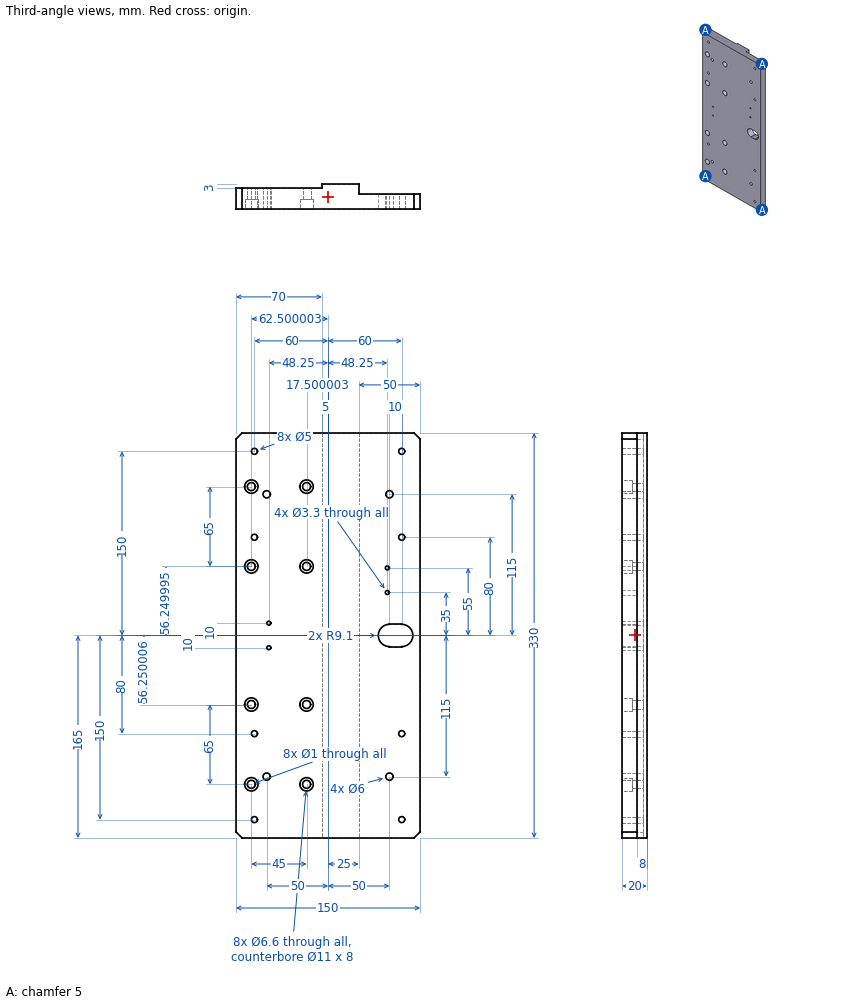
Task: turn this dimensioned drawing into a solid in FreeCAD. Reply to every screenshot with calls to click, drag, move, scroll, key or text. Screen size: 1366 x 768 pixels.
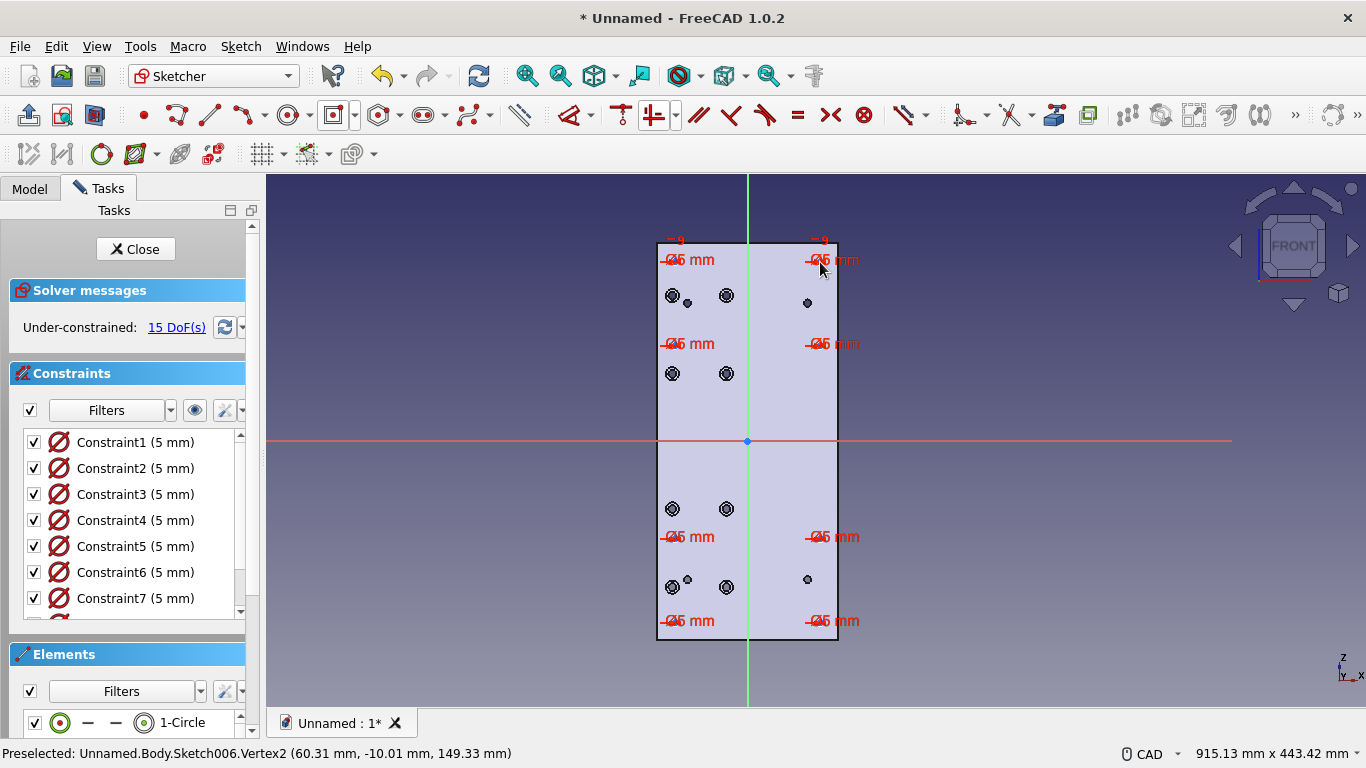
click(820, 262)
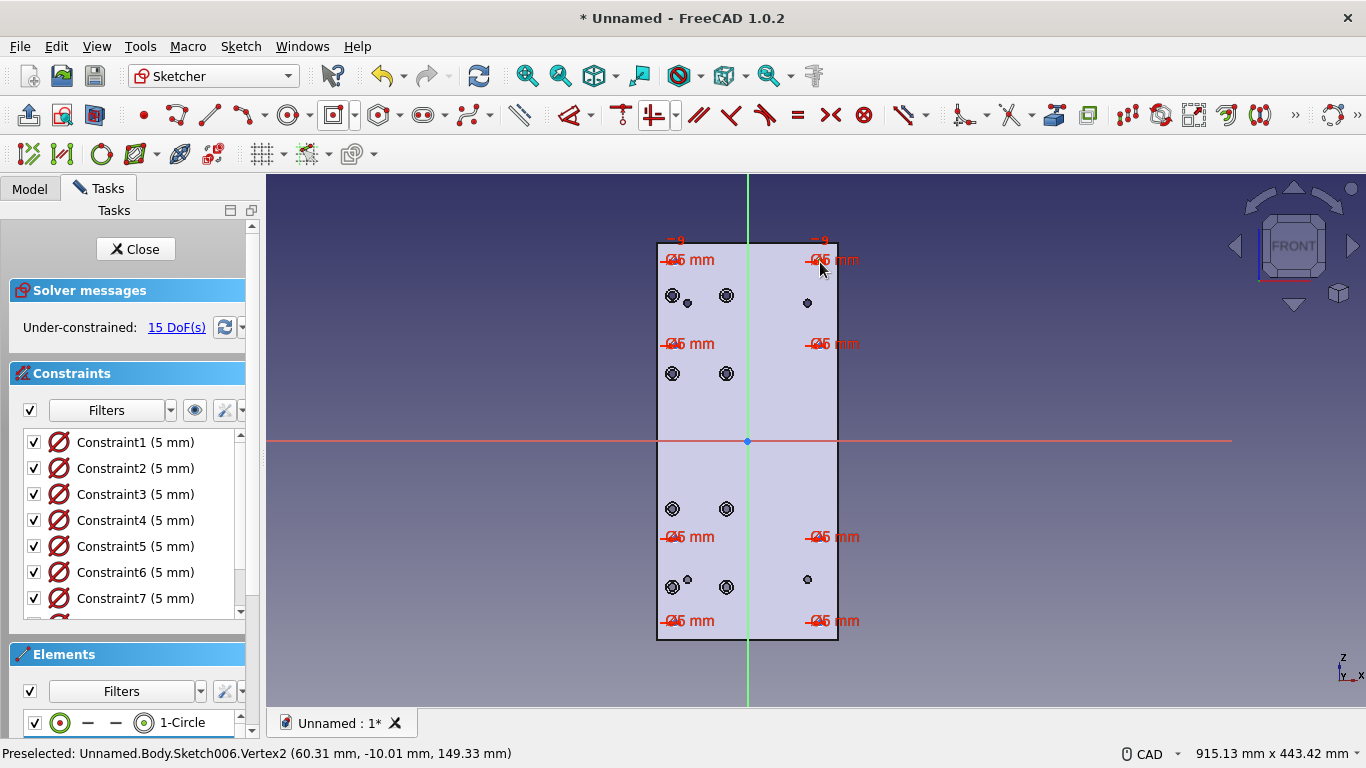
click(820, 346)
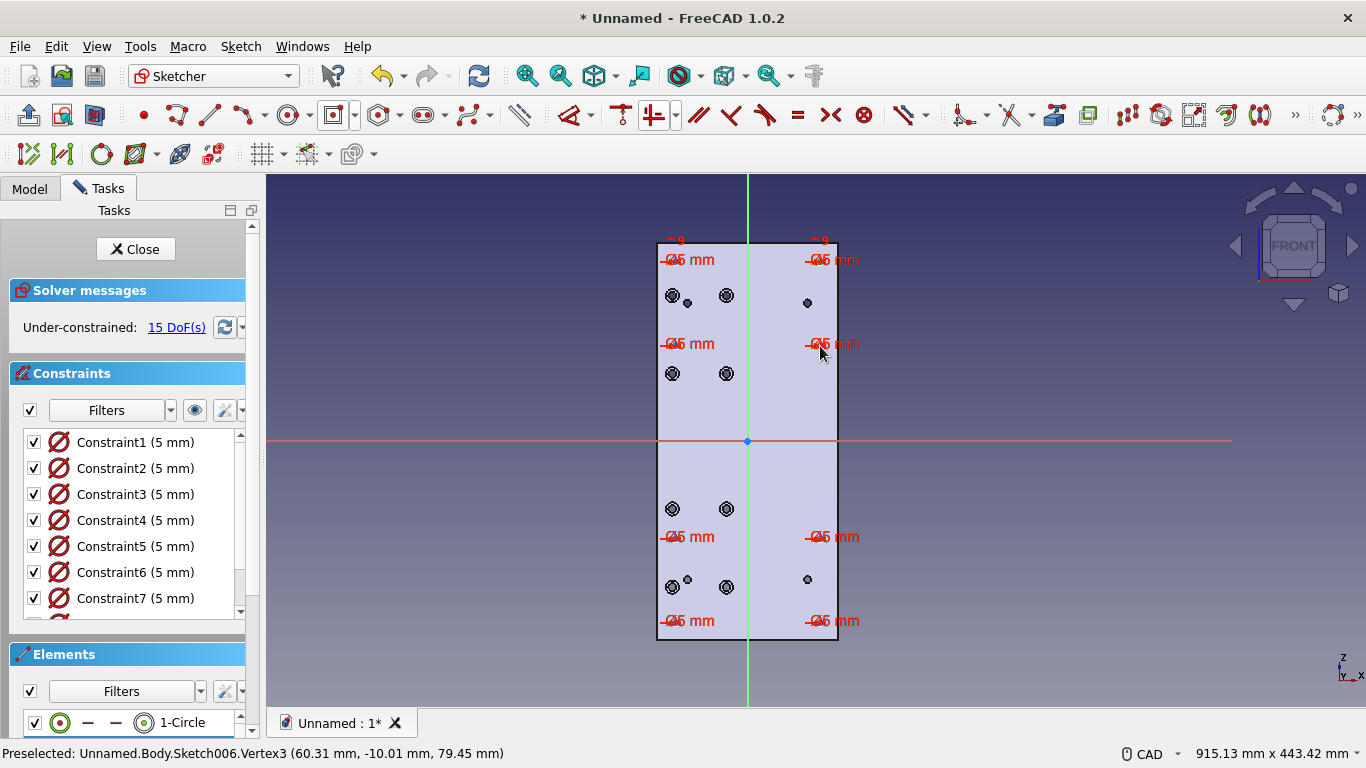
key(v)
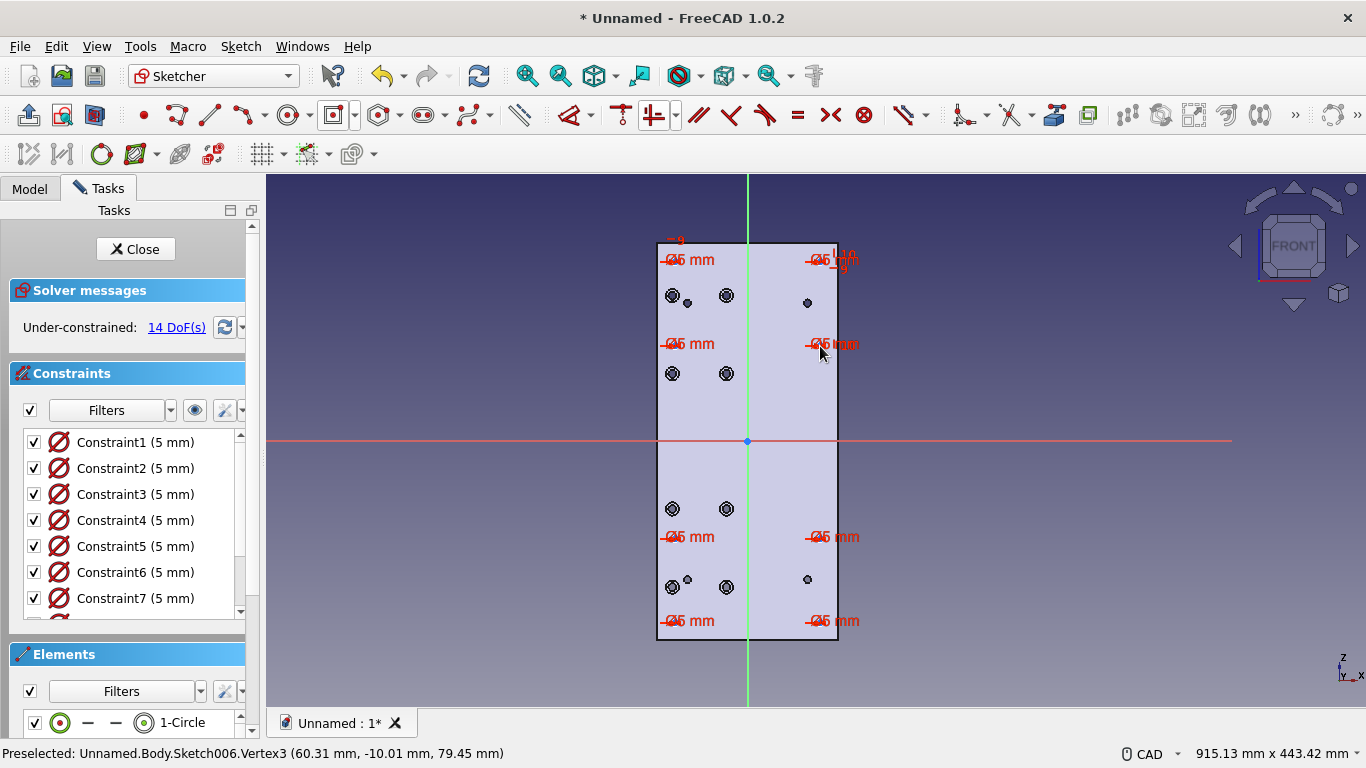
click(675, 262)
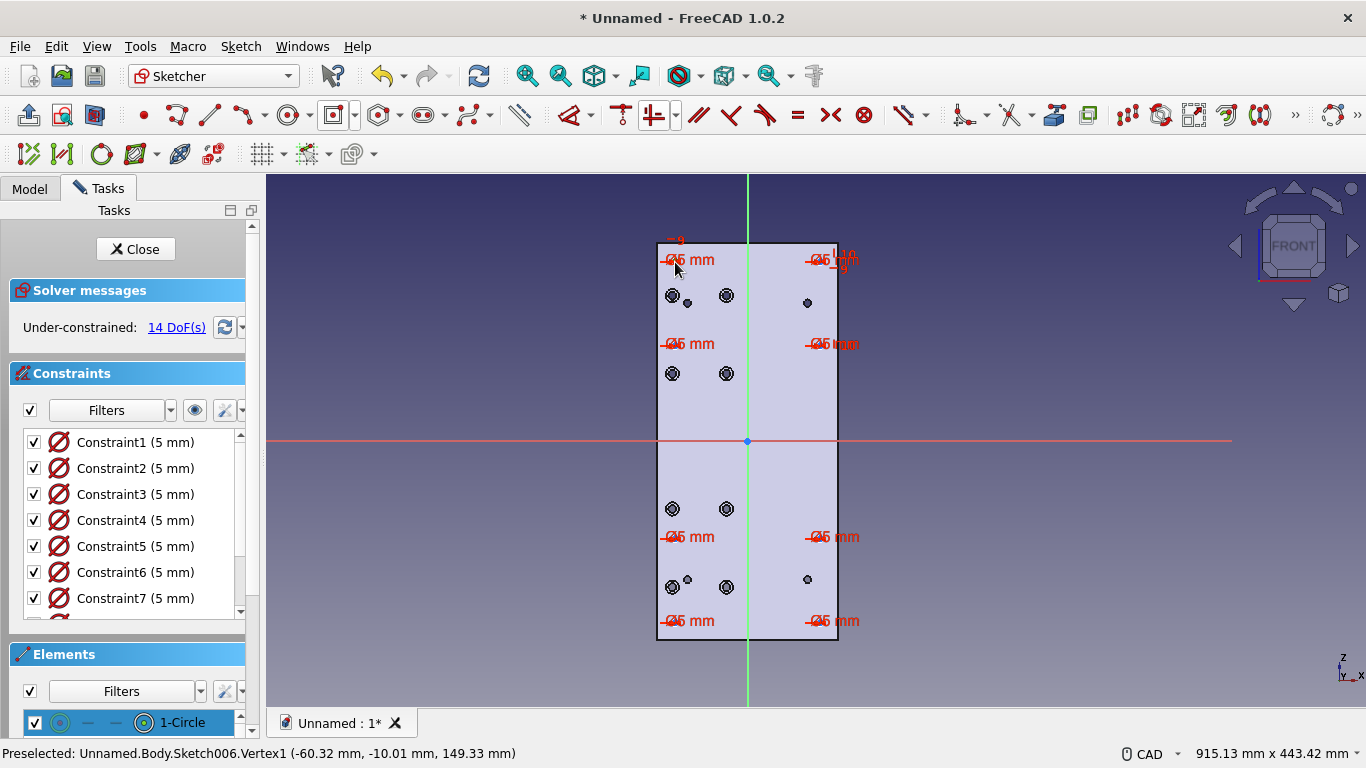
click(675, 346)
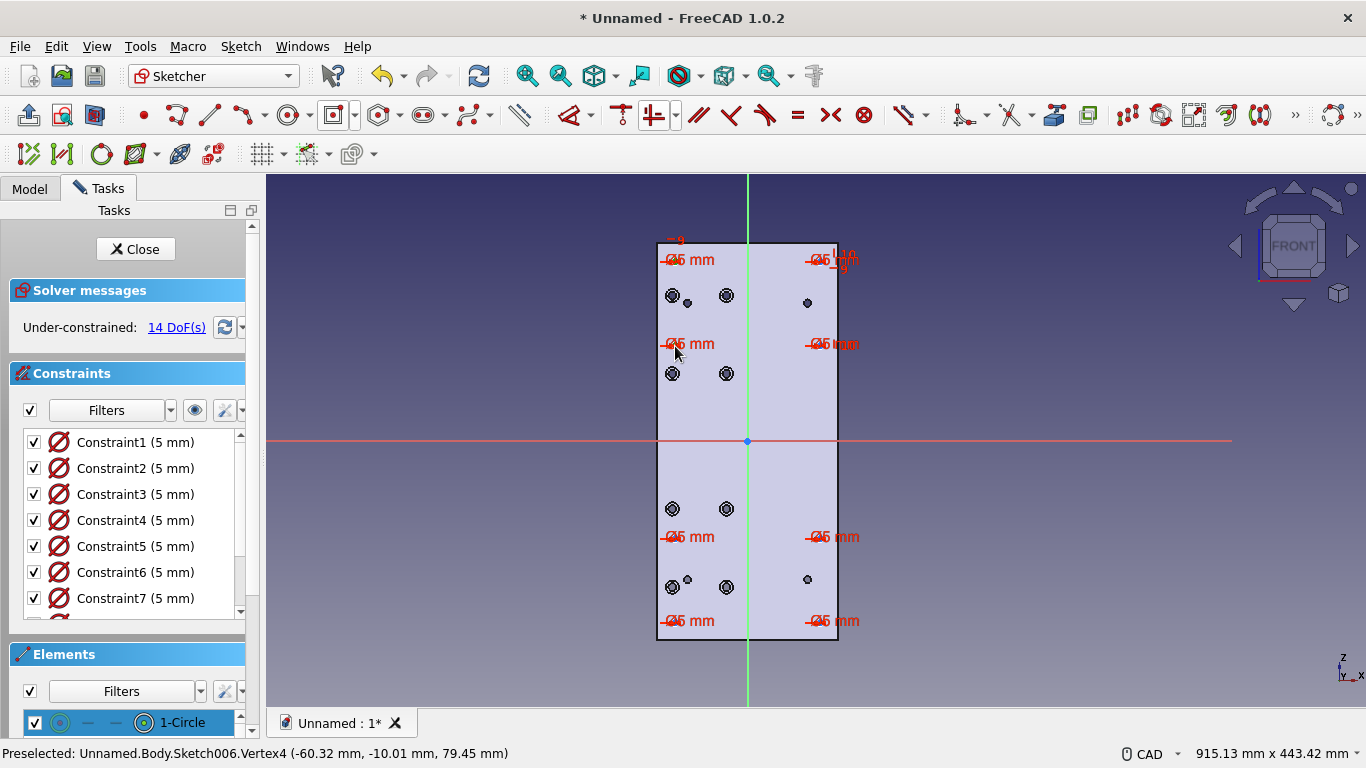
click(676, 116)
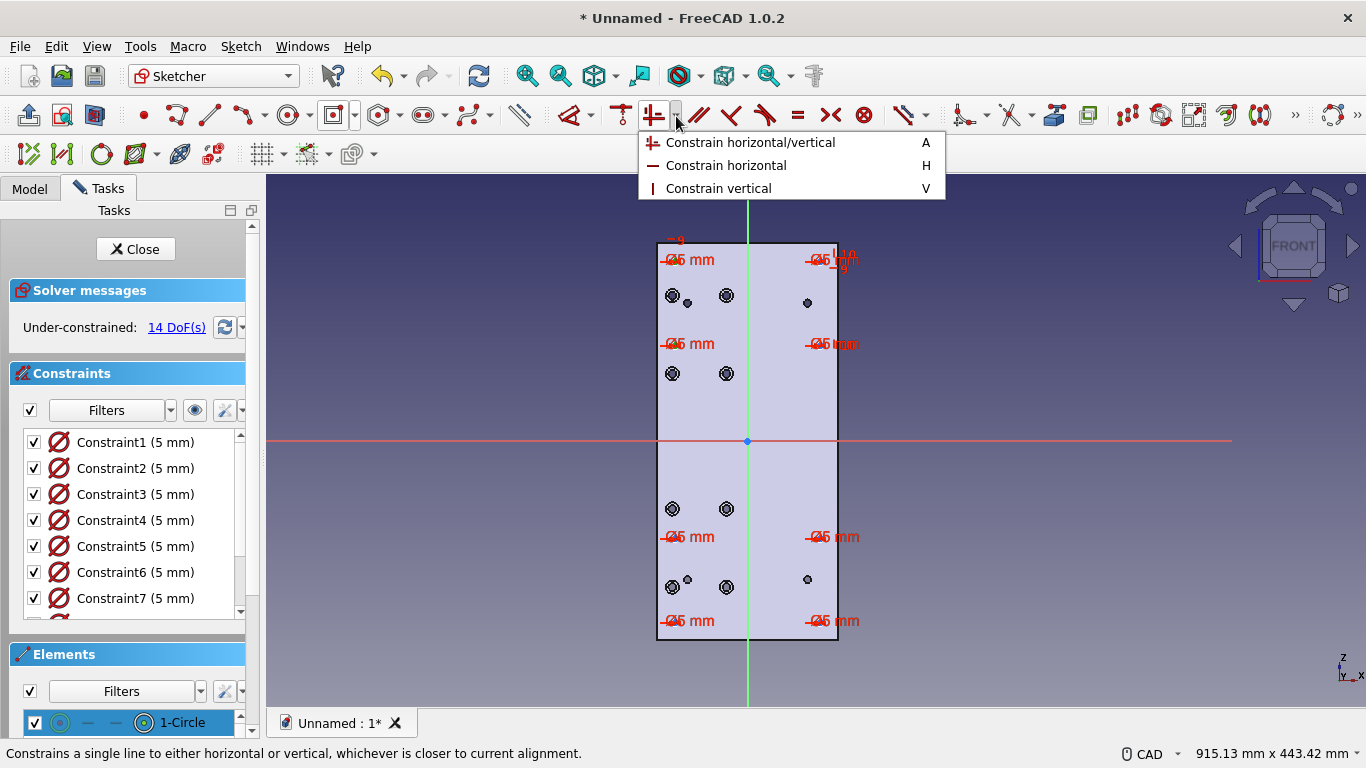
click(792, 188)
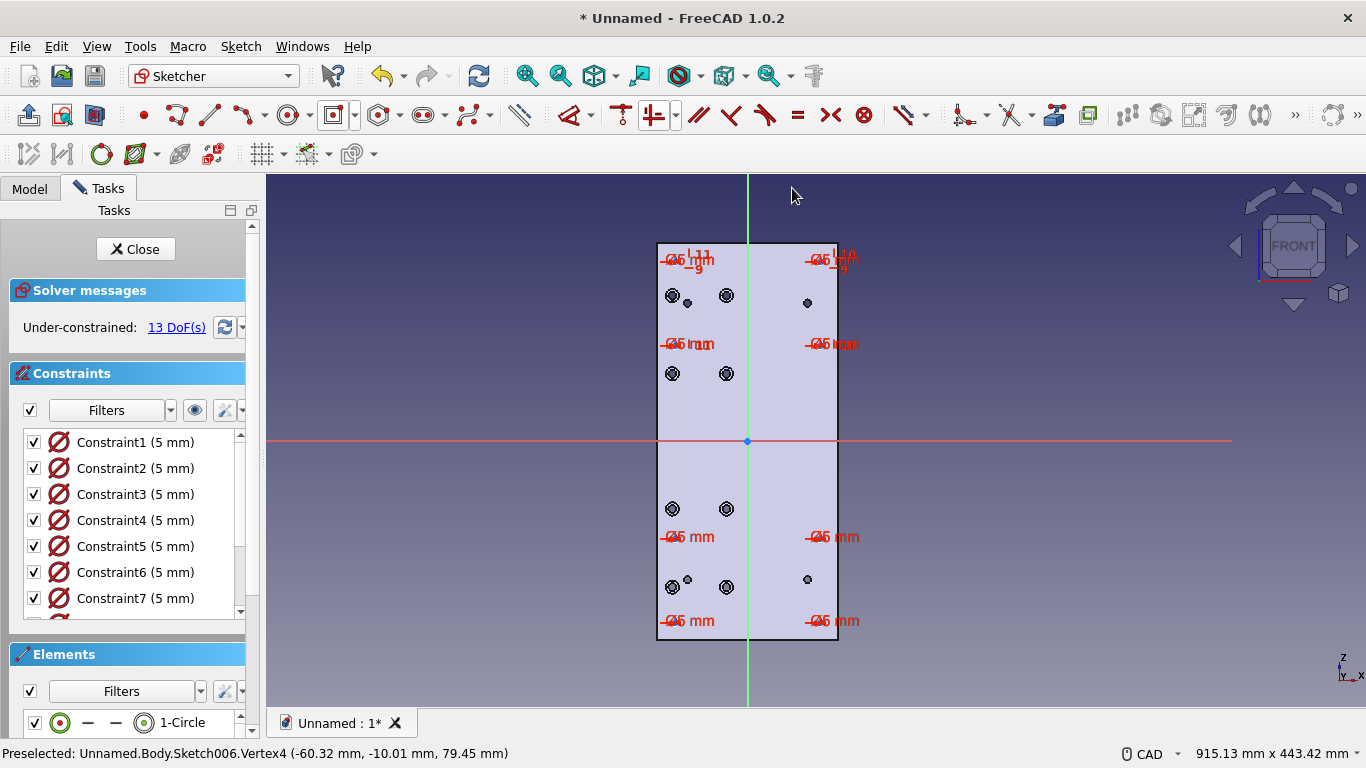
click(820, 346)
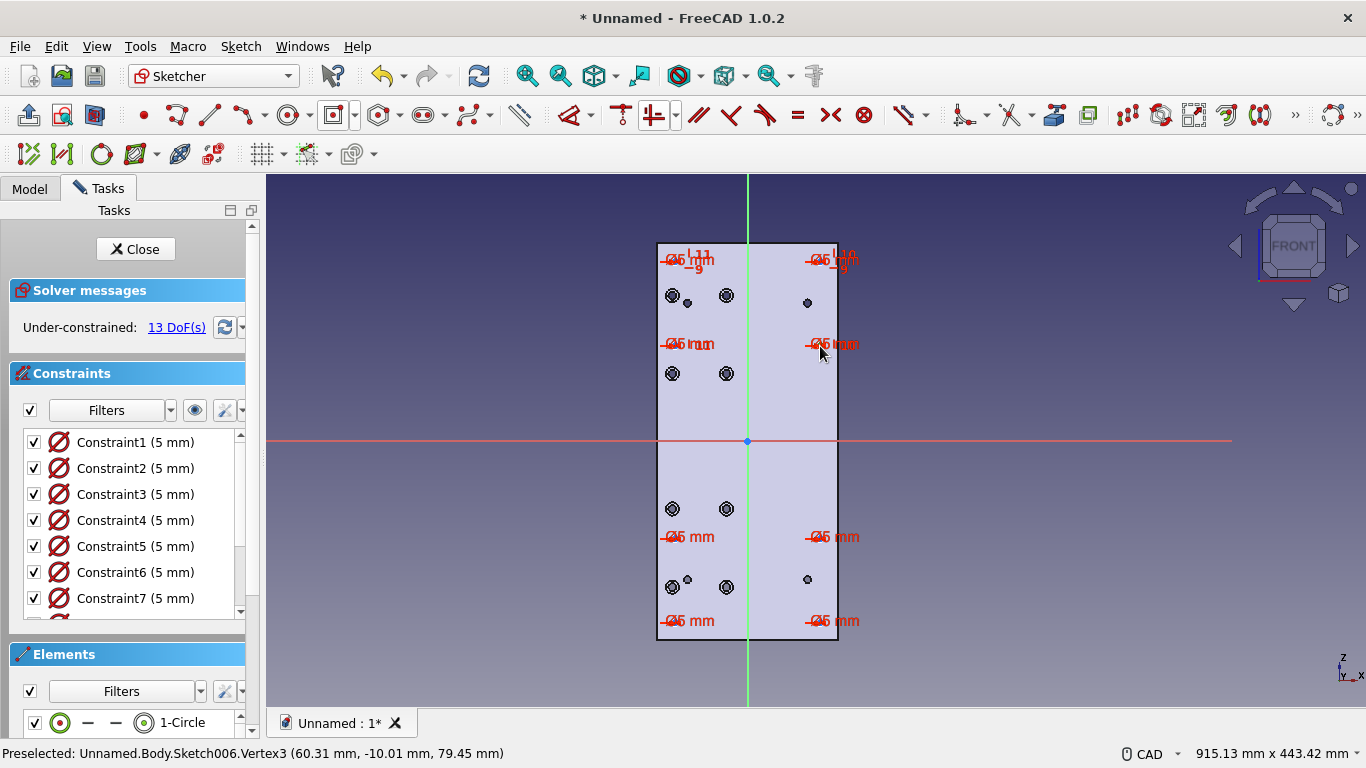
click(675, 346)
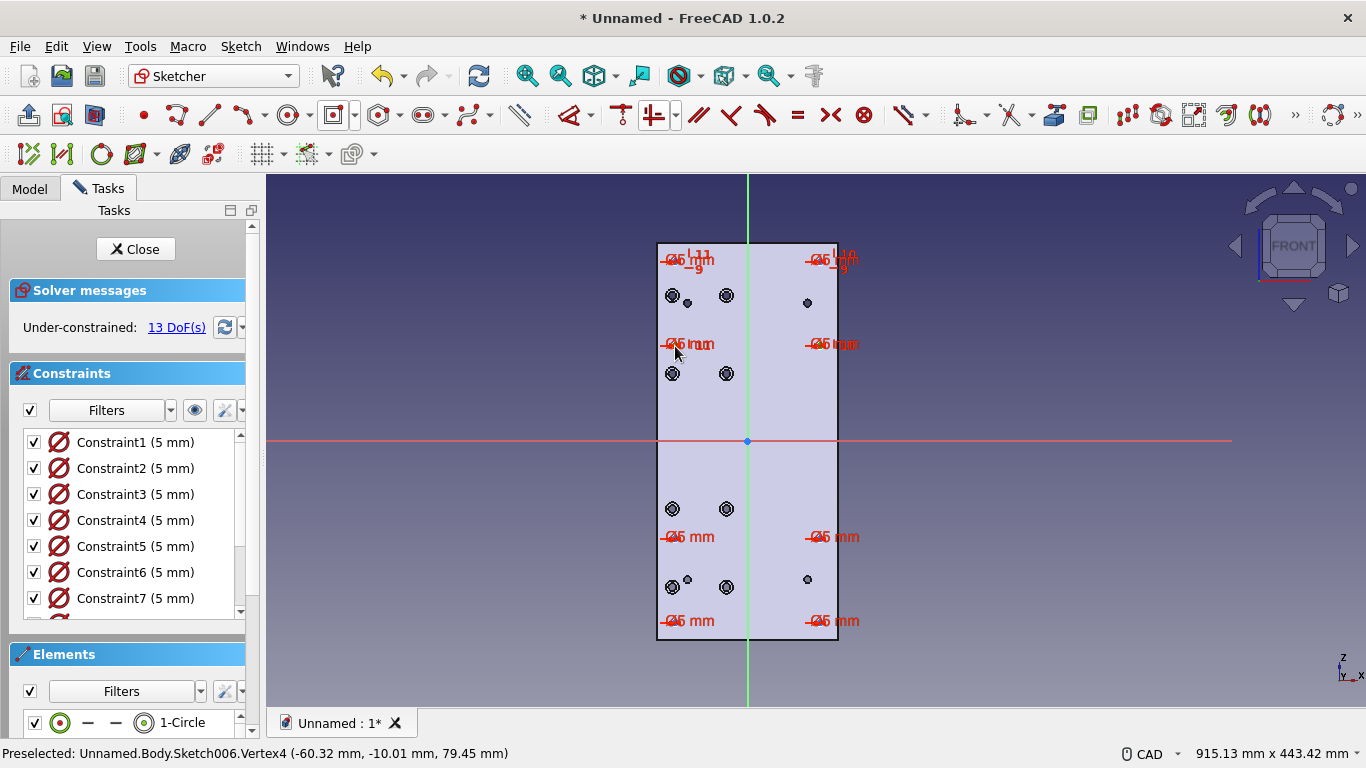
click(676, 116)